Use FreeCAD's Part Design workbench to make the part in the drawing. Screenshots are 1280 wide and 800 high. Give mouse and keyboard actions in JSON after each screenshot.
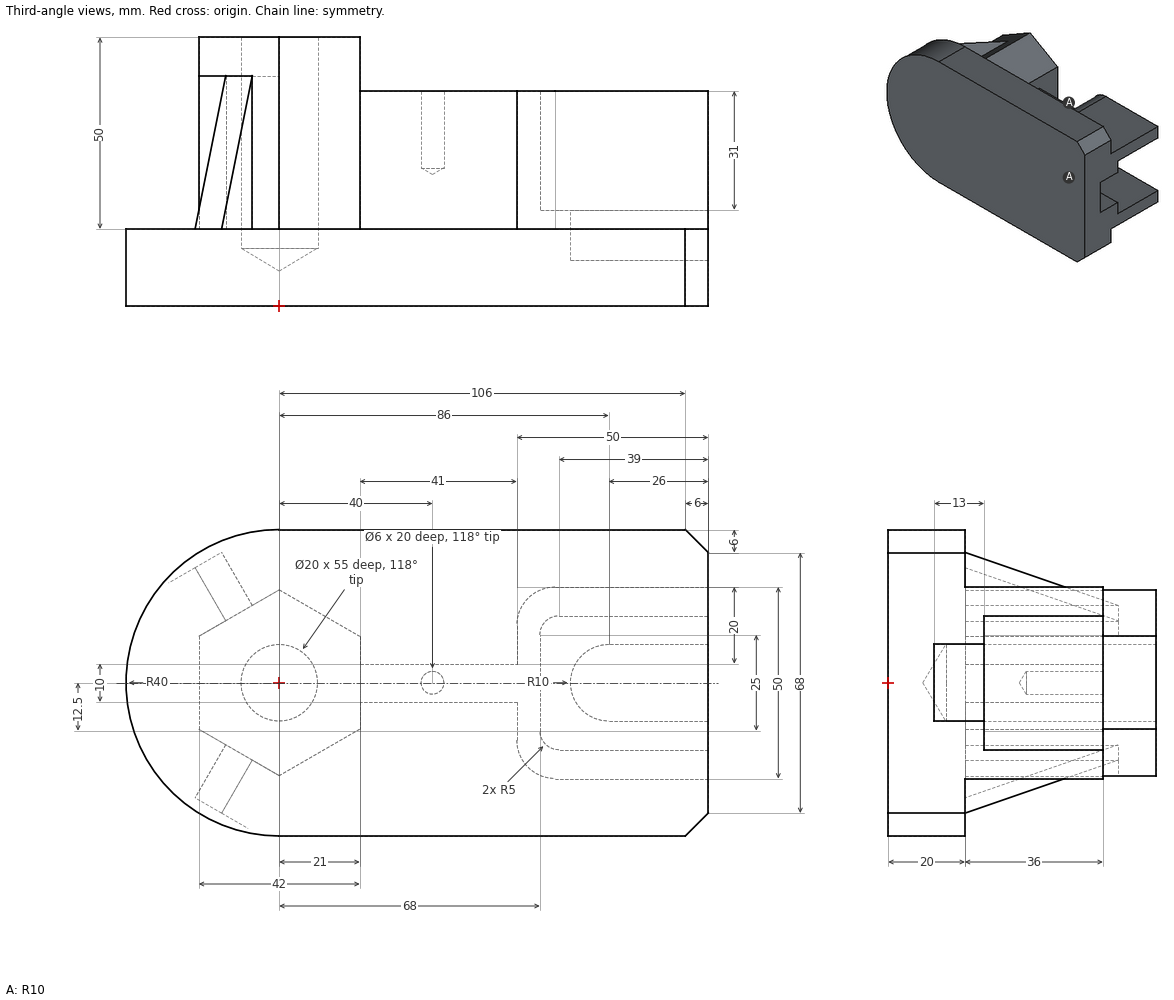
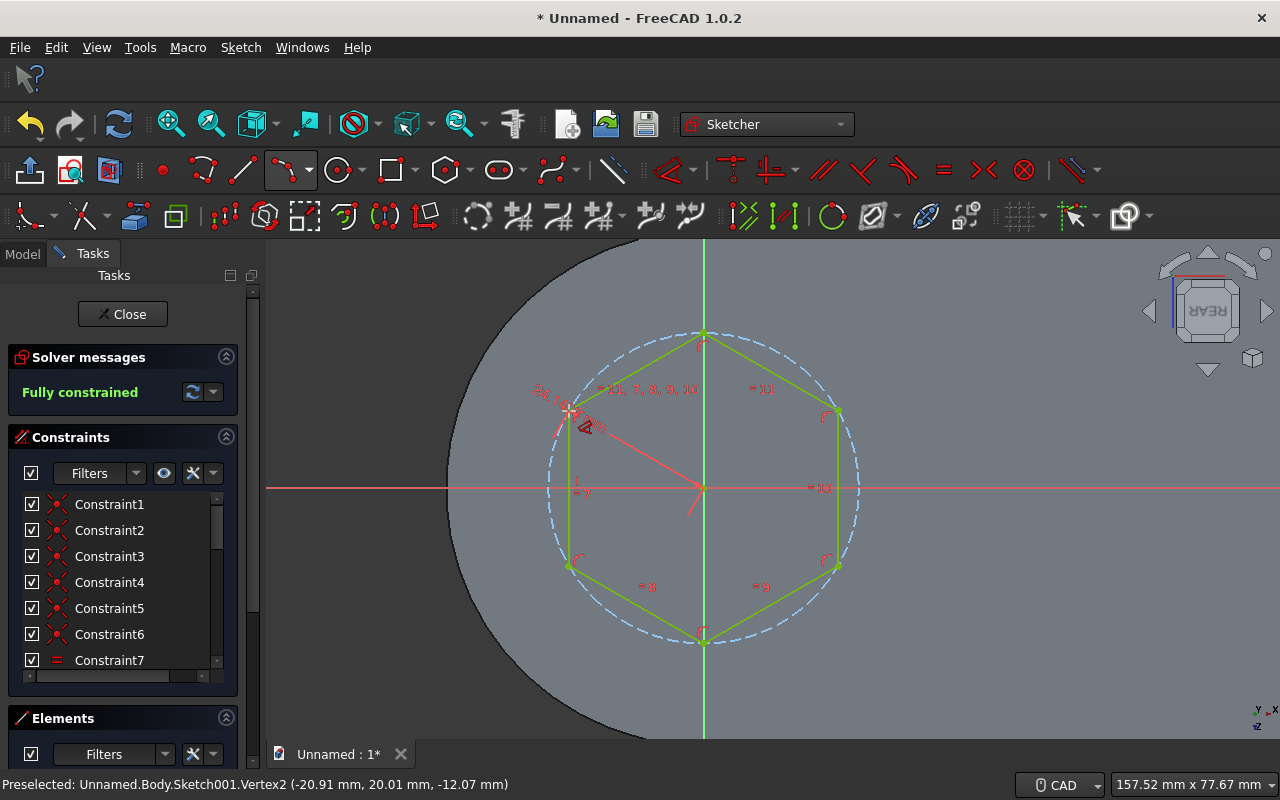
{"action": "left_click", "coordinate": [838, 566]}
{"action": "left_click", "coordinate": [642, 648]}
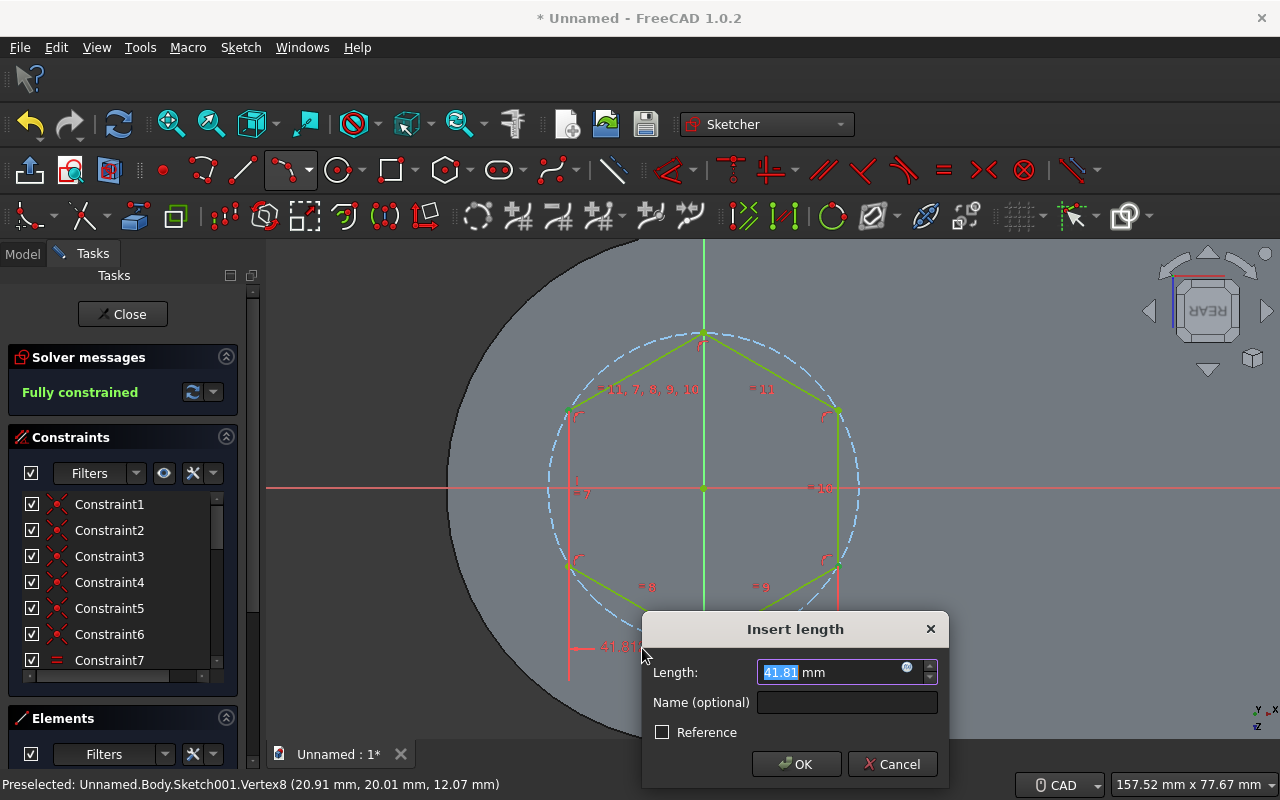
{"action": "type", "text": "42"}
{"action": "key", "text": "Return"}
{"action": "key", "text": "Escape"}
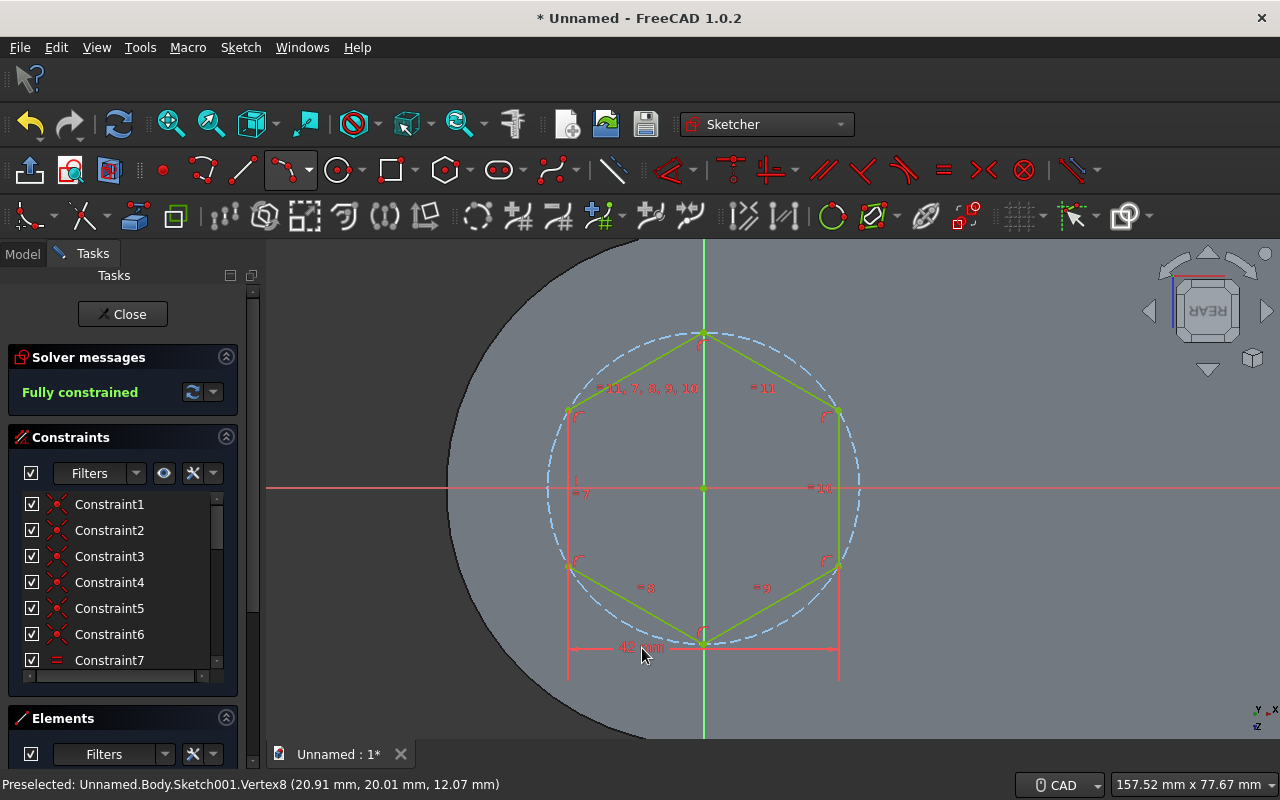
{"action": "left_click", "coordinate": [123, 314]}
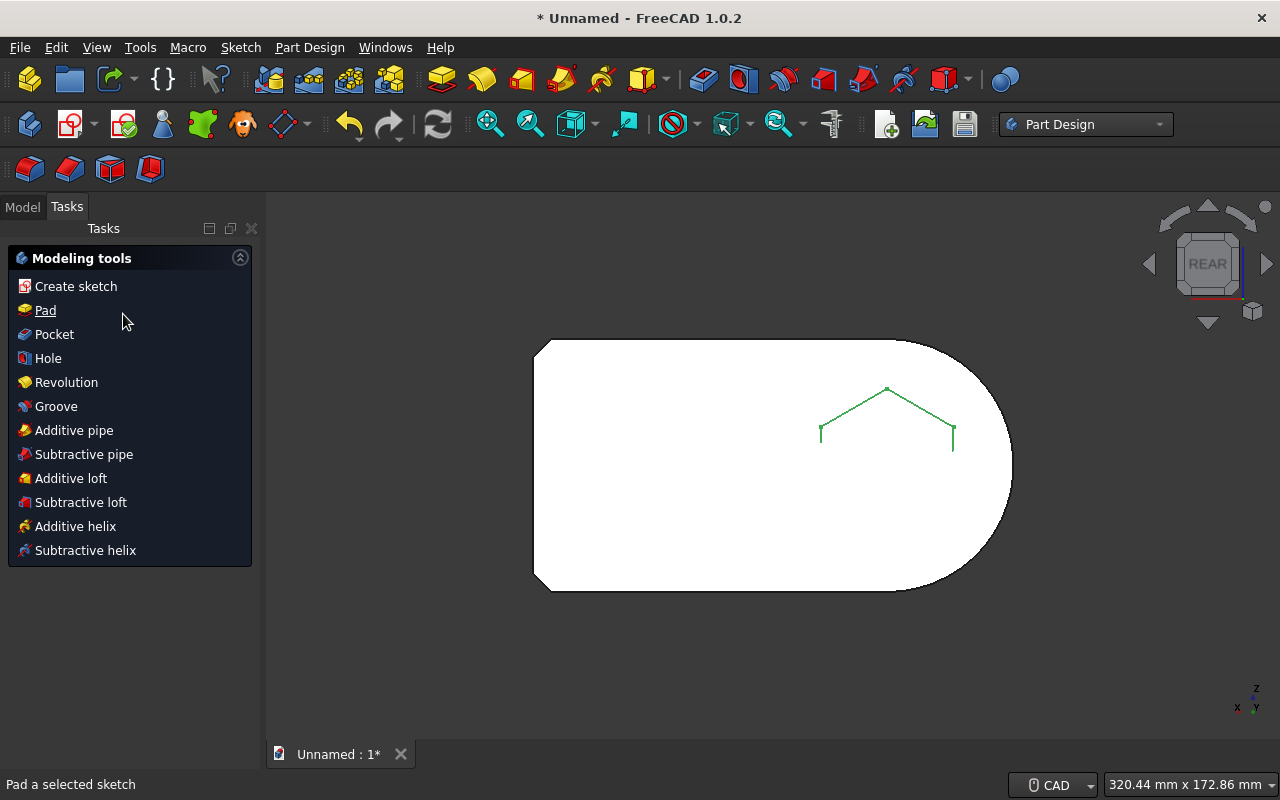
{"action": "left_click", "coordinate": [442, 80]}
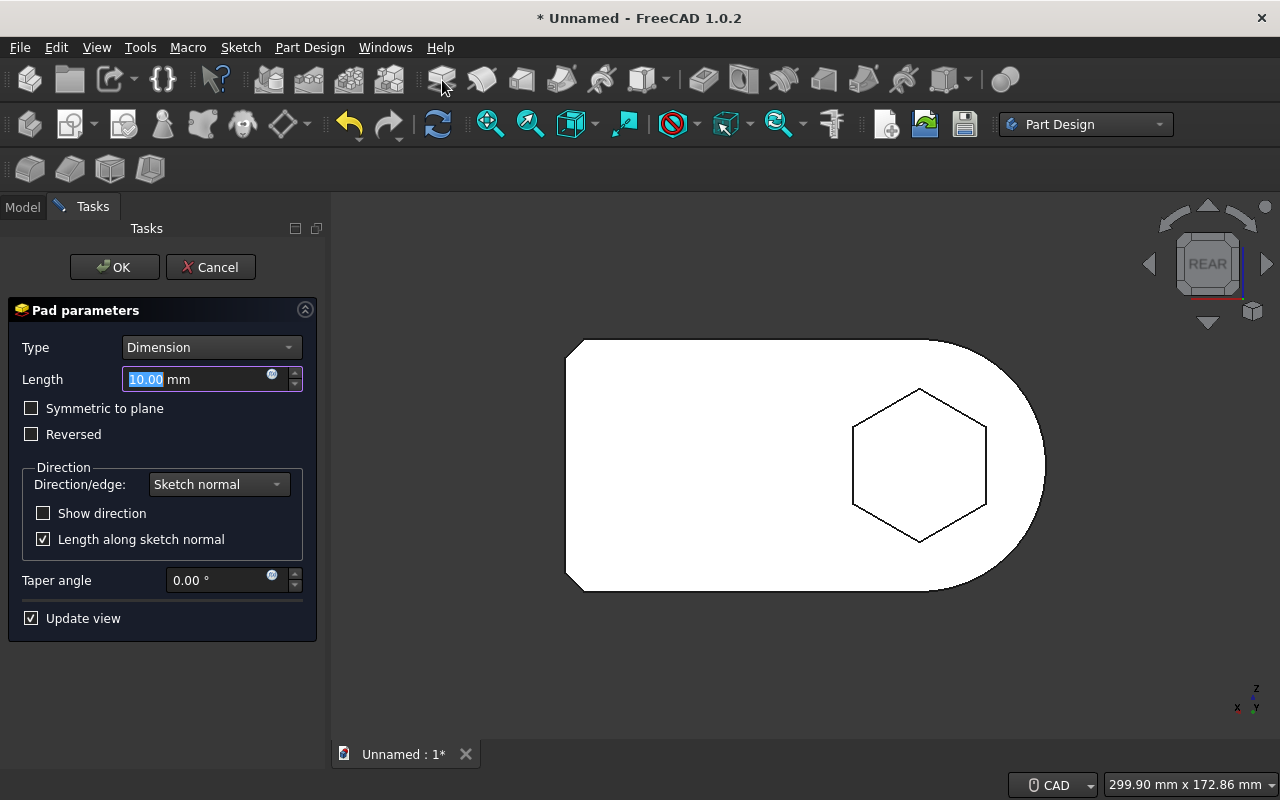
{"action": "type", "text": "50"}
{"action": "key", "text": "Tab"}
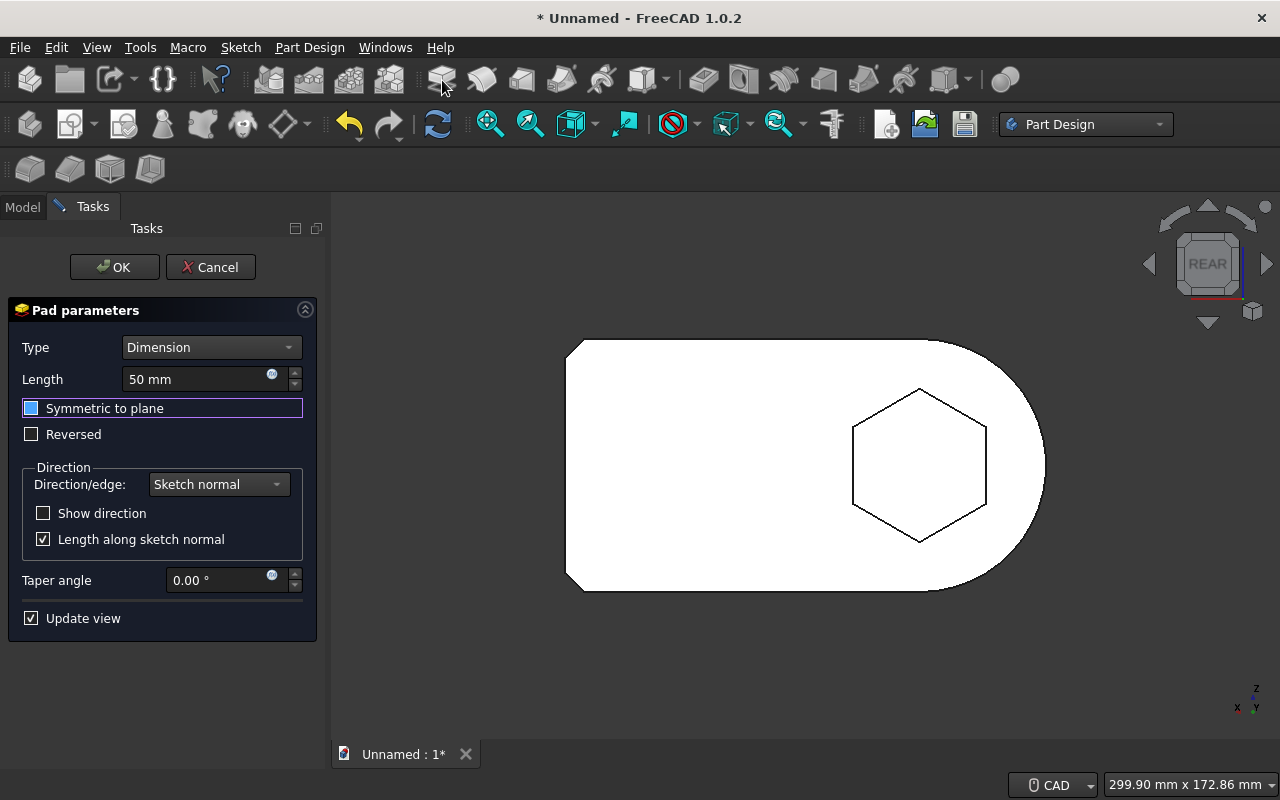
{"action": "left_click", "coordinate": [115, 267]}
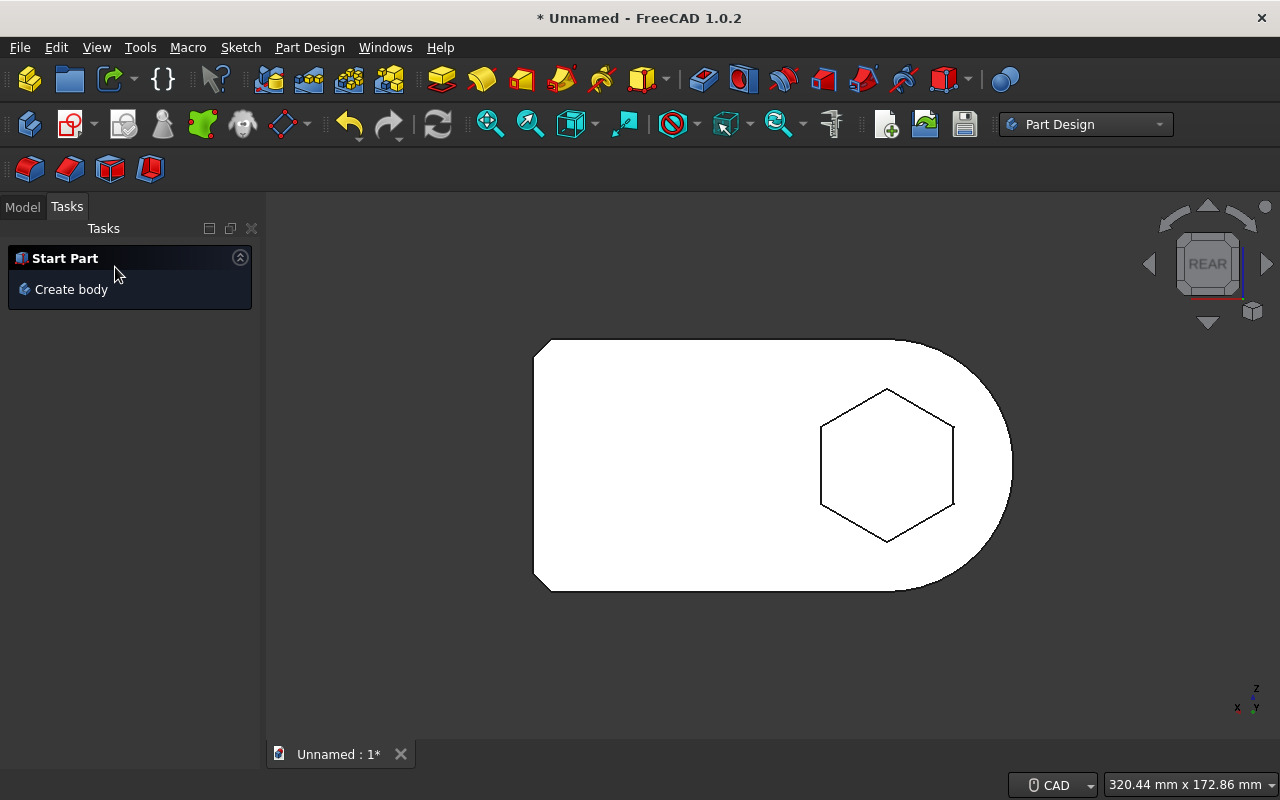
{"action": "key", "text": "2"}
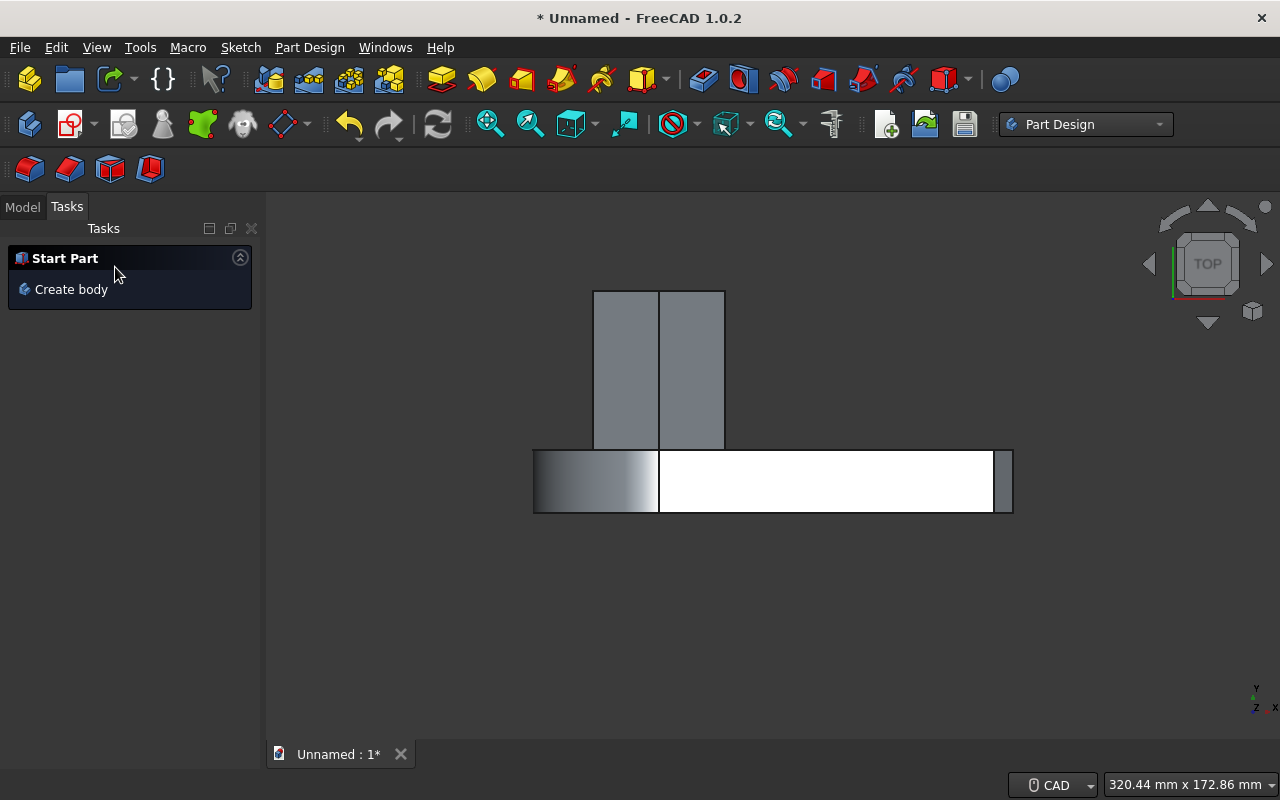
{"action": "left_click", "coordinate": [626, 347]}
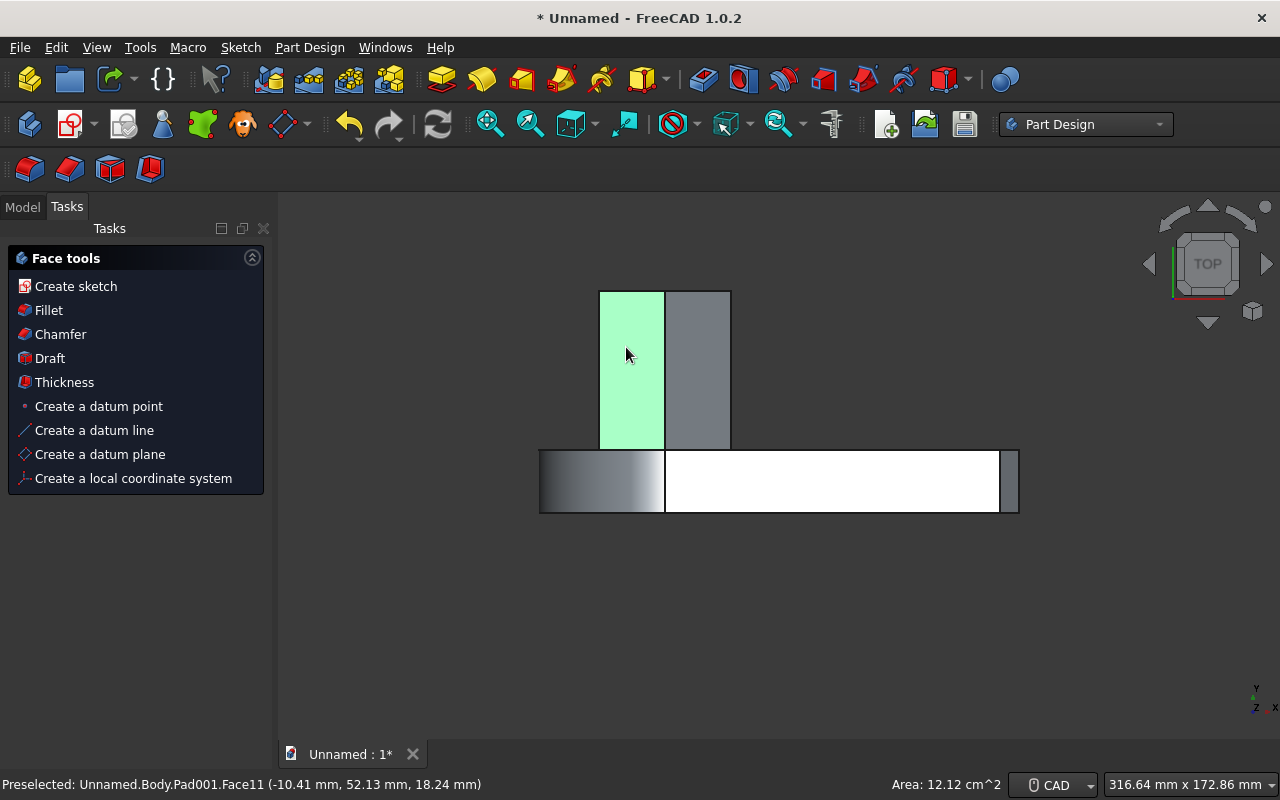
{"action": "left_click", "coordinate": [70, 124]}